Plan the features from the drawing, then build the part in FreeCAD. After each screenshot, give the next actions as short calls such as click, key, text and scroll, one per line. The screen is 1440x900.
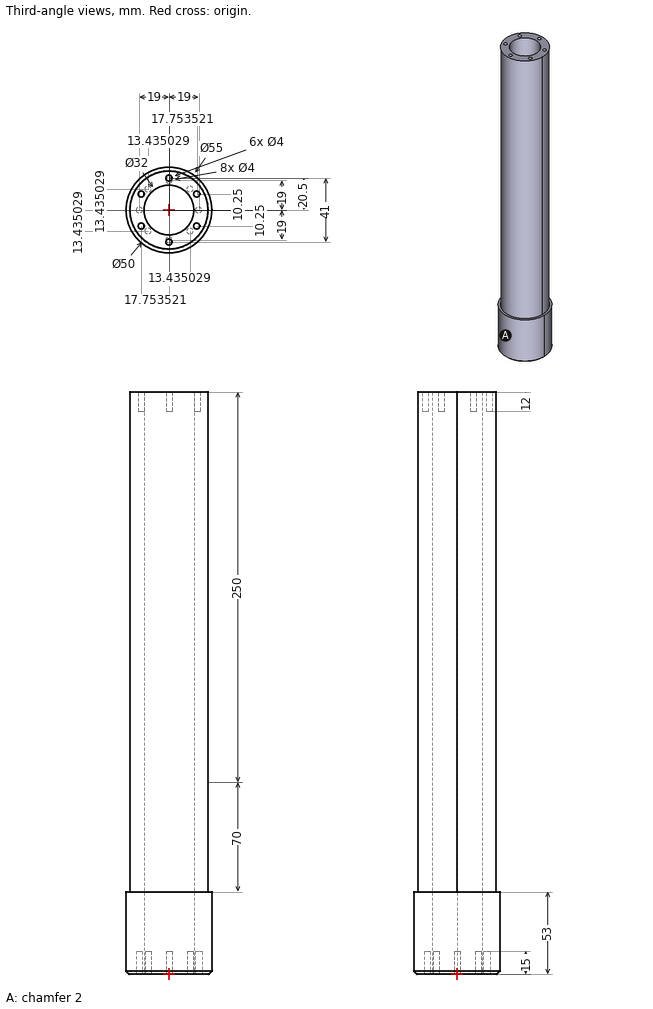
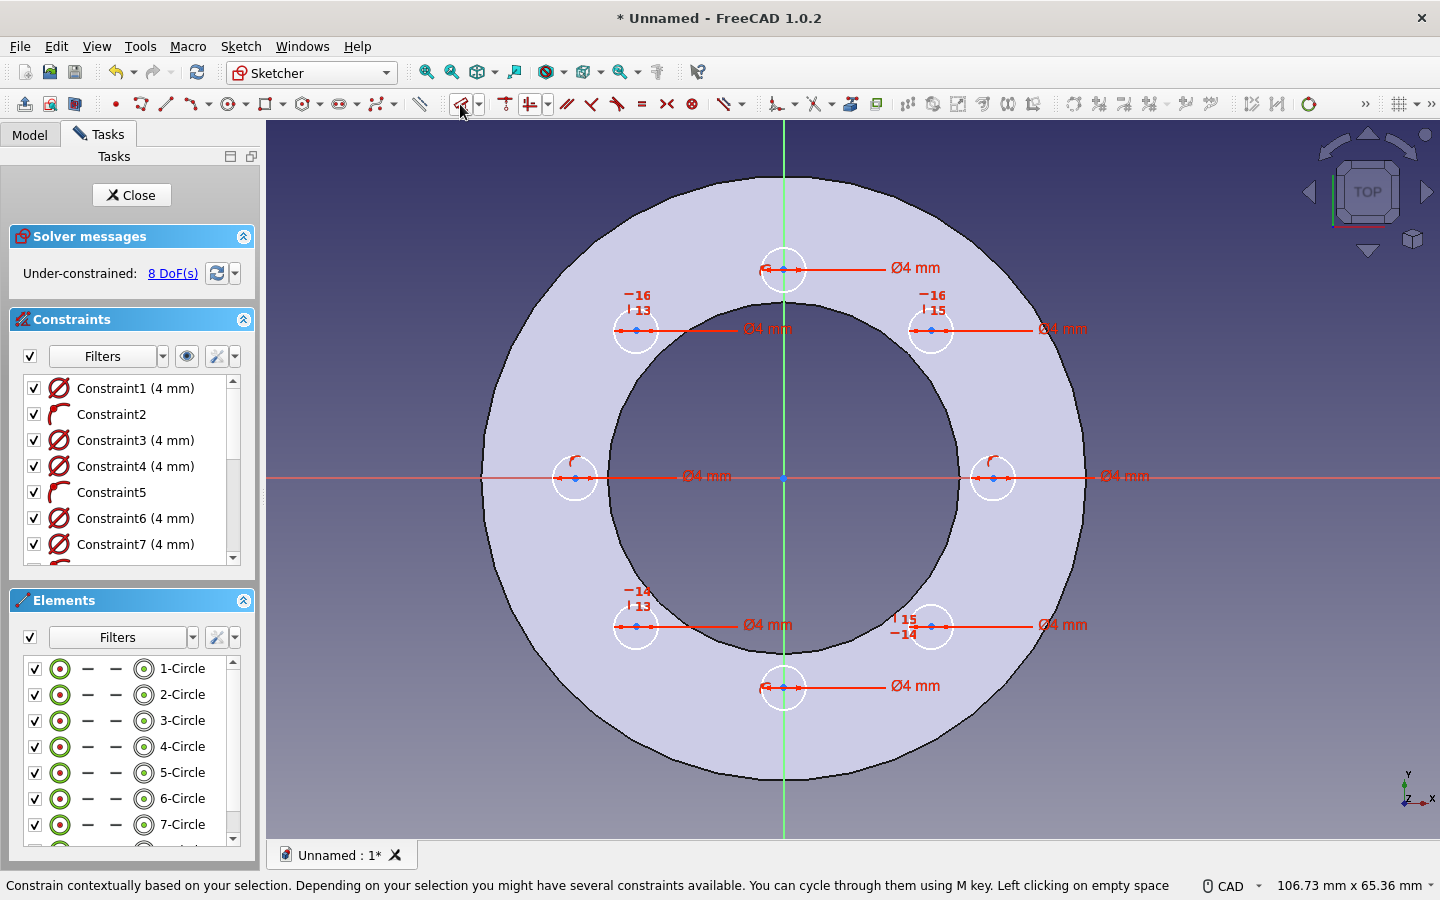
click(784, 270)
click(818, 374)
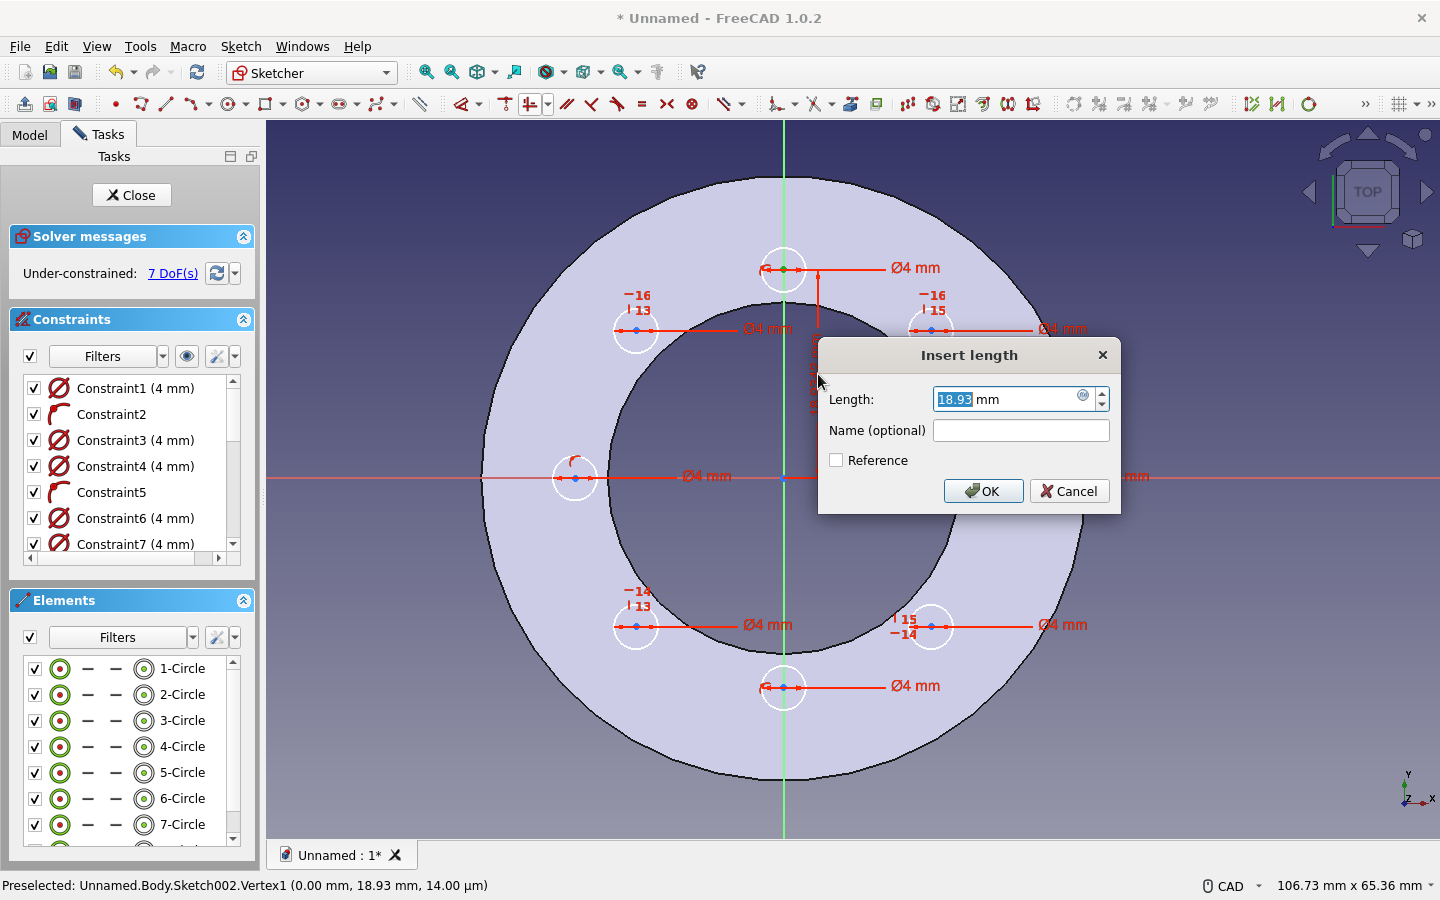
text(19)
key(Return)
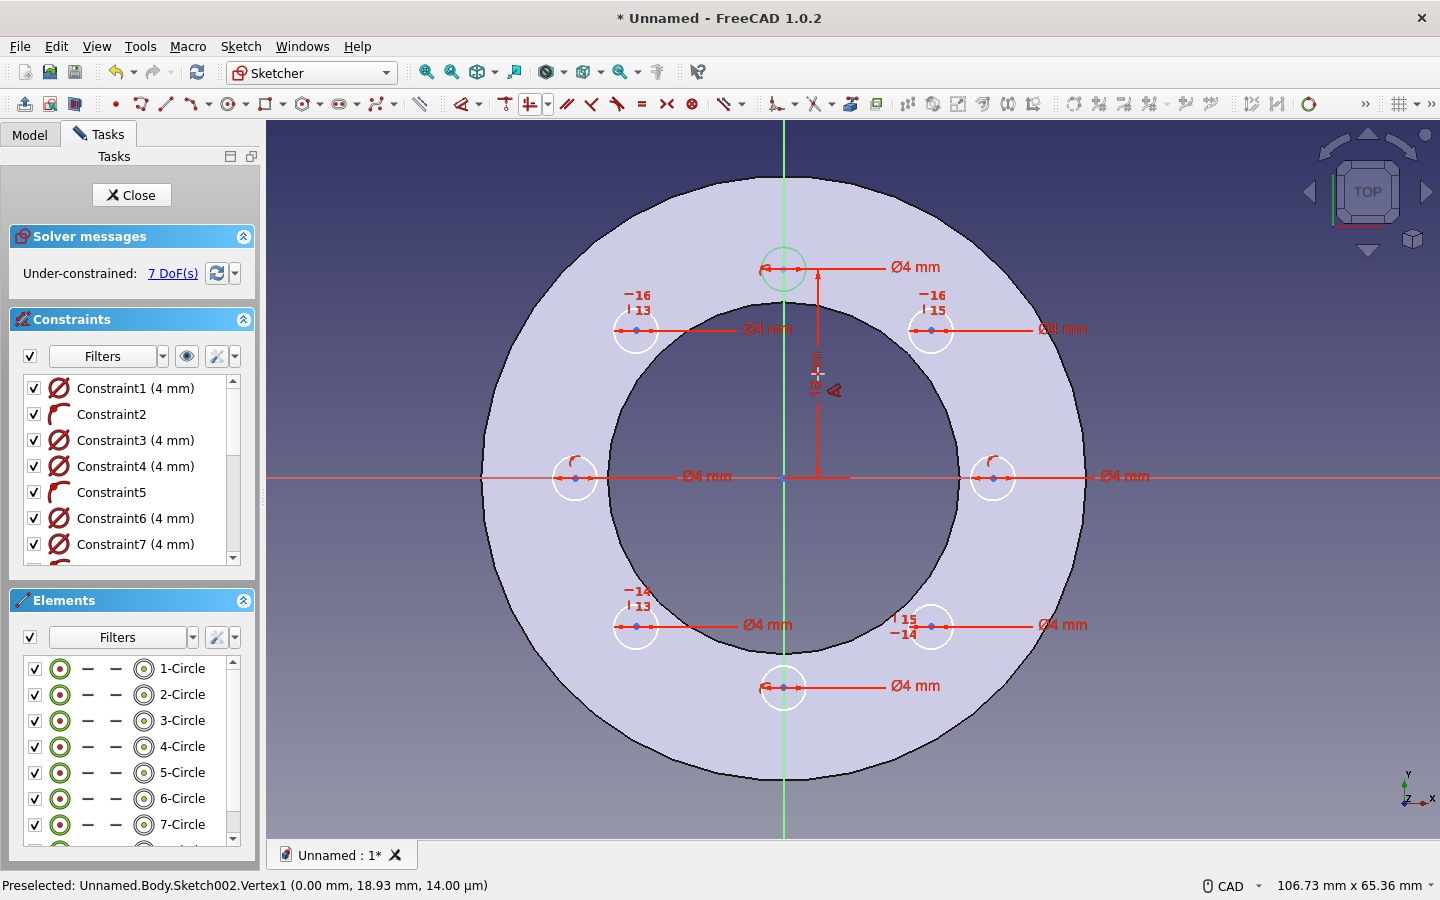
click(575, 478)
click(679, 512)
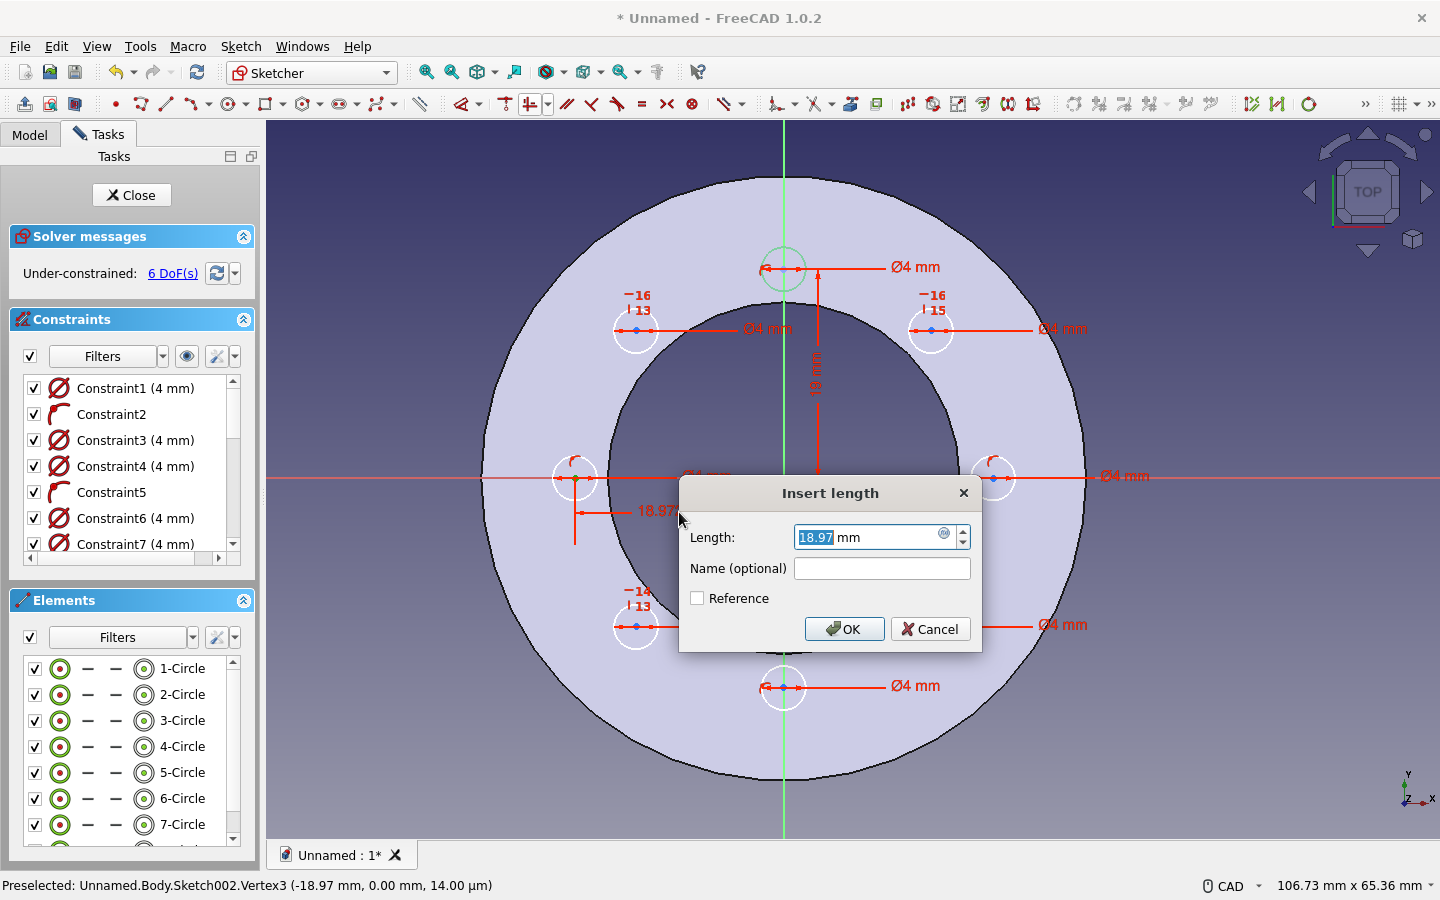
text(19)
key(Return)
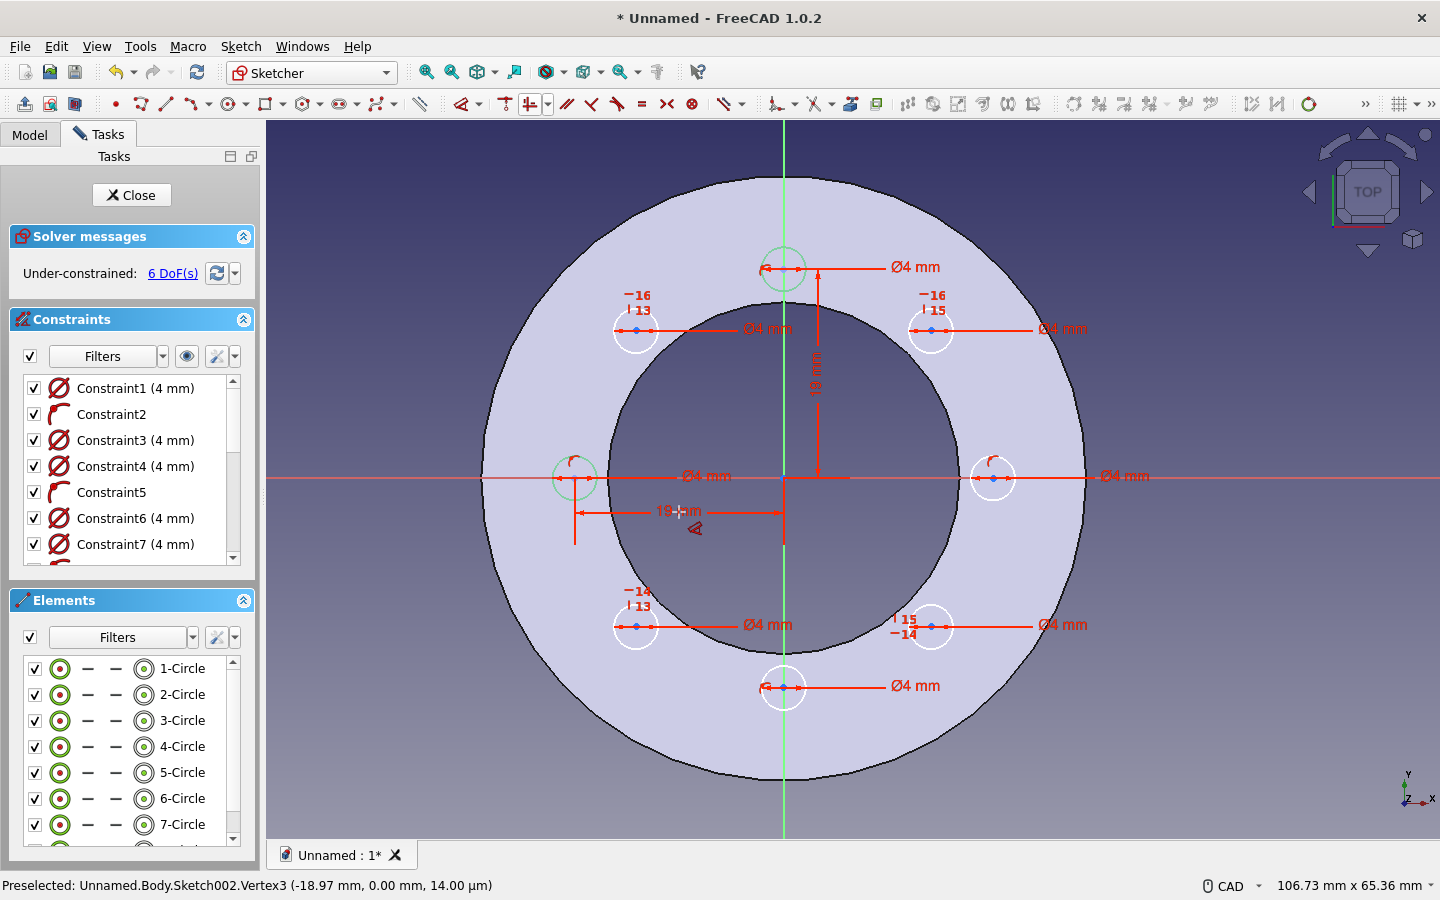
click(784, 688)
click(818, 583)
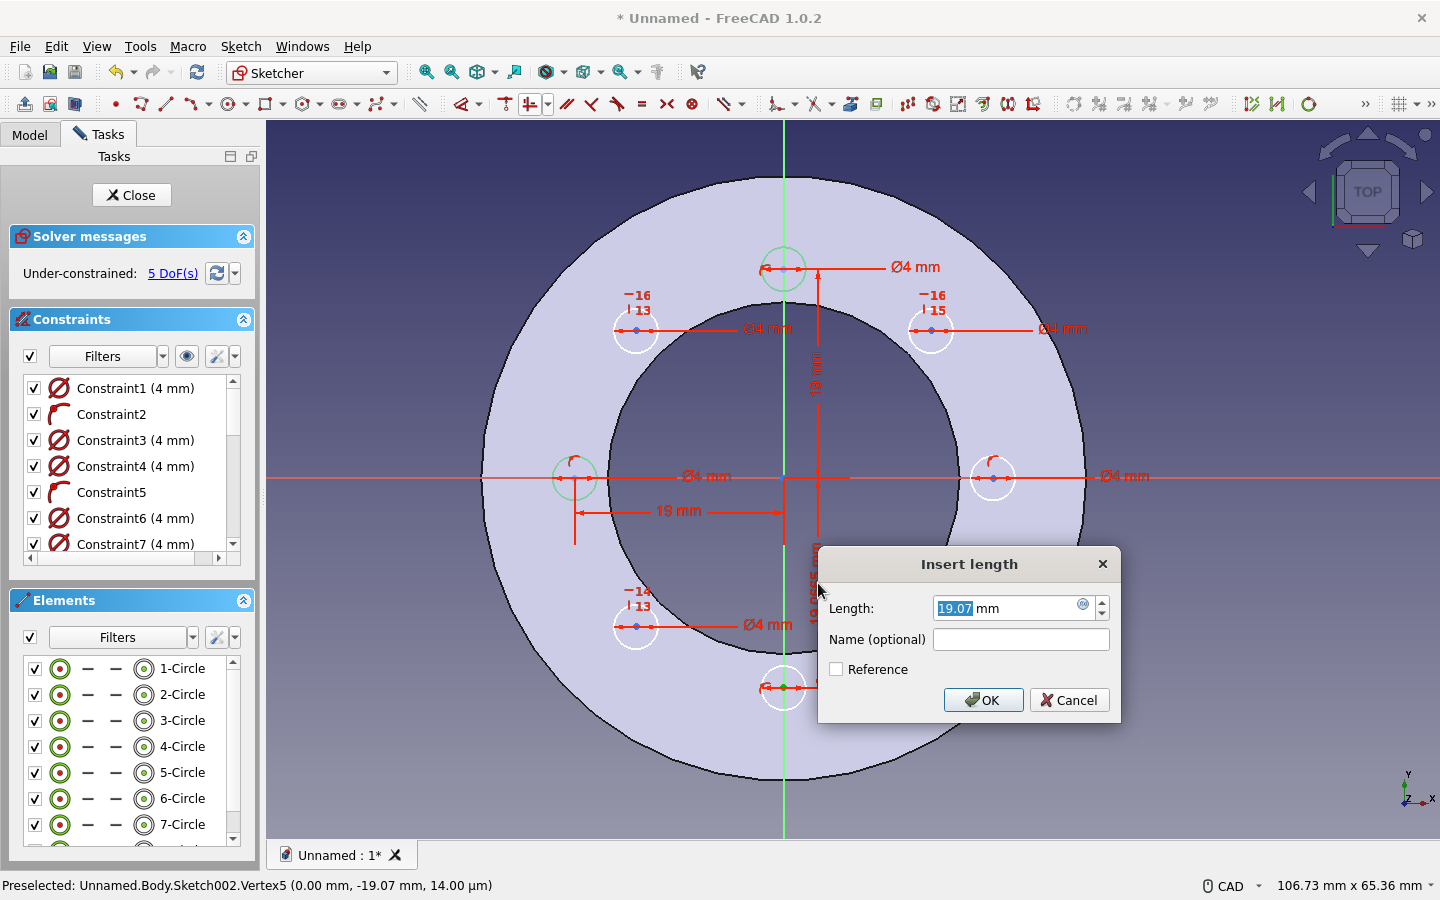
text(19)
key(Return)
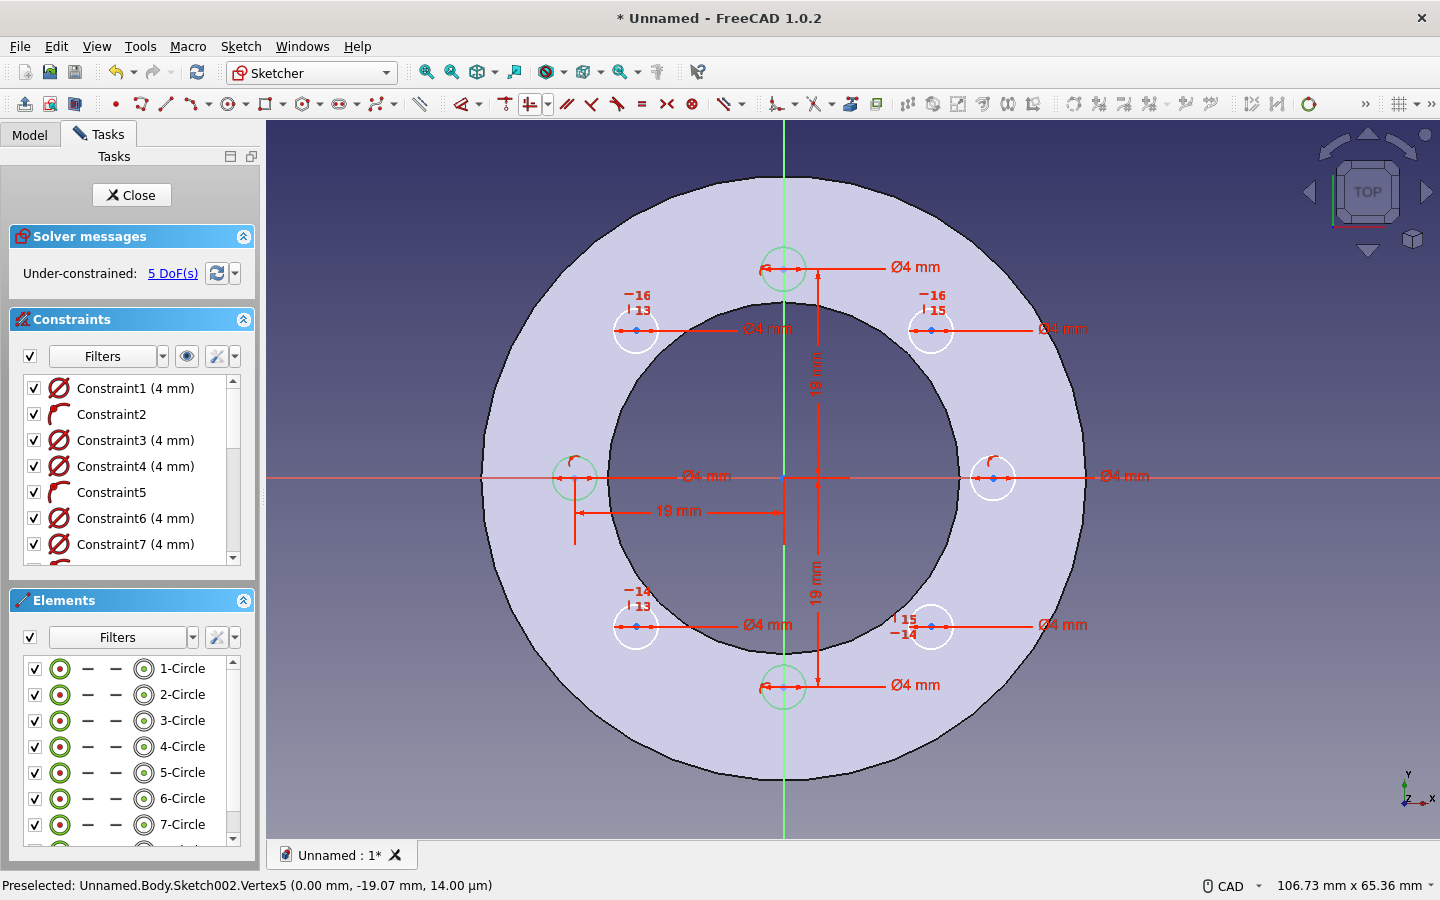
click(993, 478)
click(888, 512)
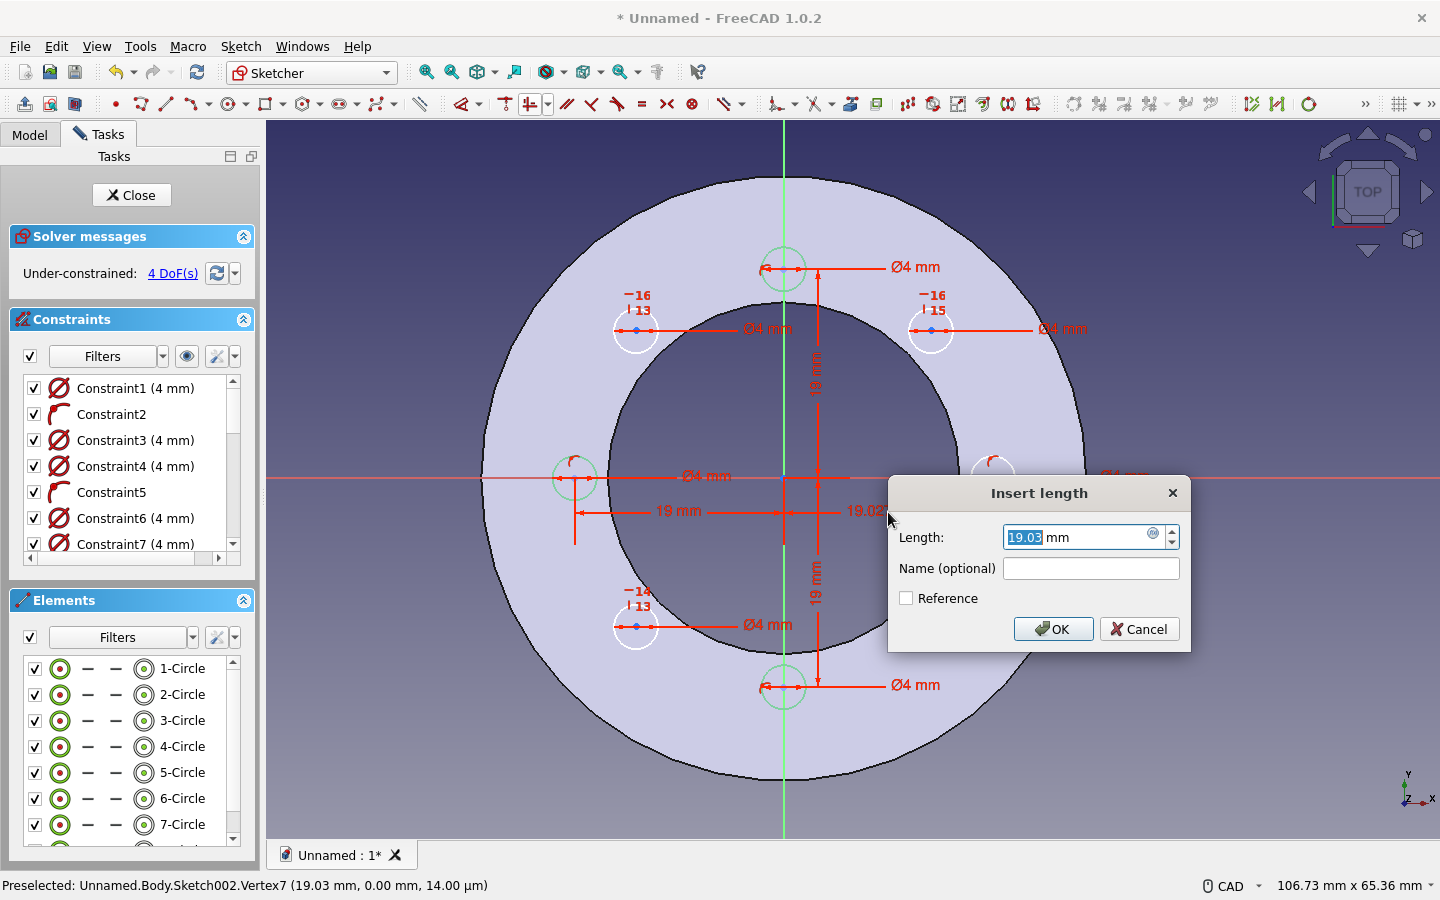
text(19)
key(Return)